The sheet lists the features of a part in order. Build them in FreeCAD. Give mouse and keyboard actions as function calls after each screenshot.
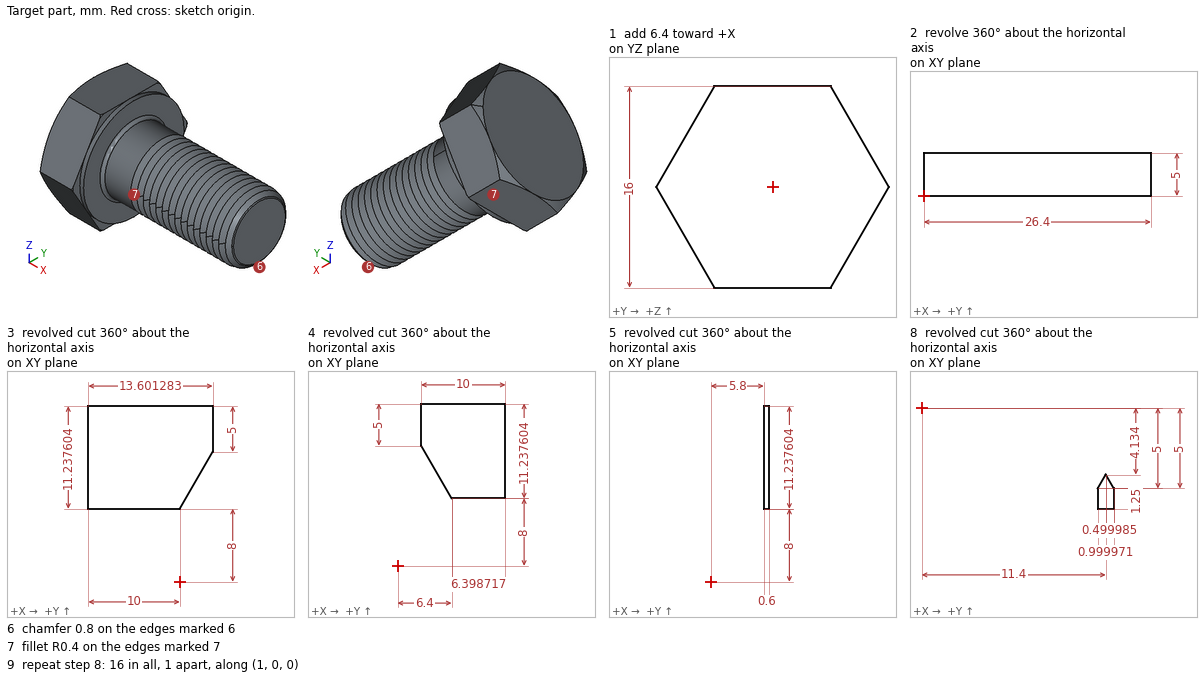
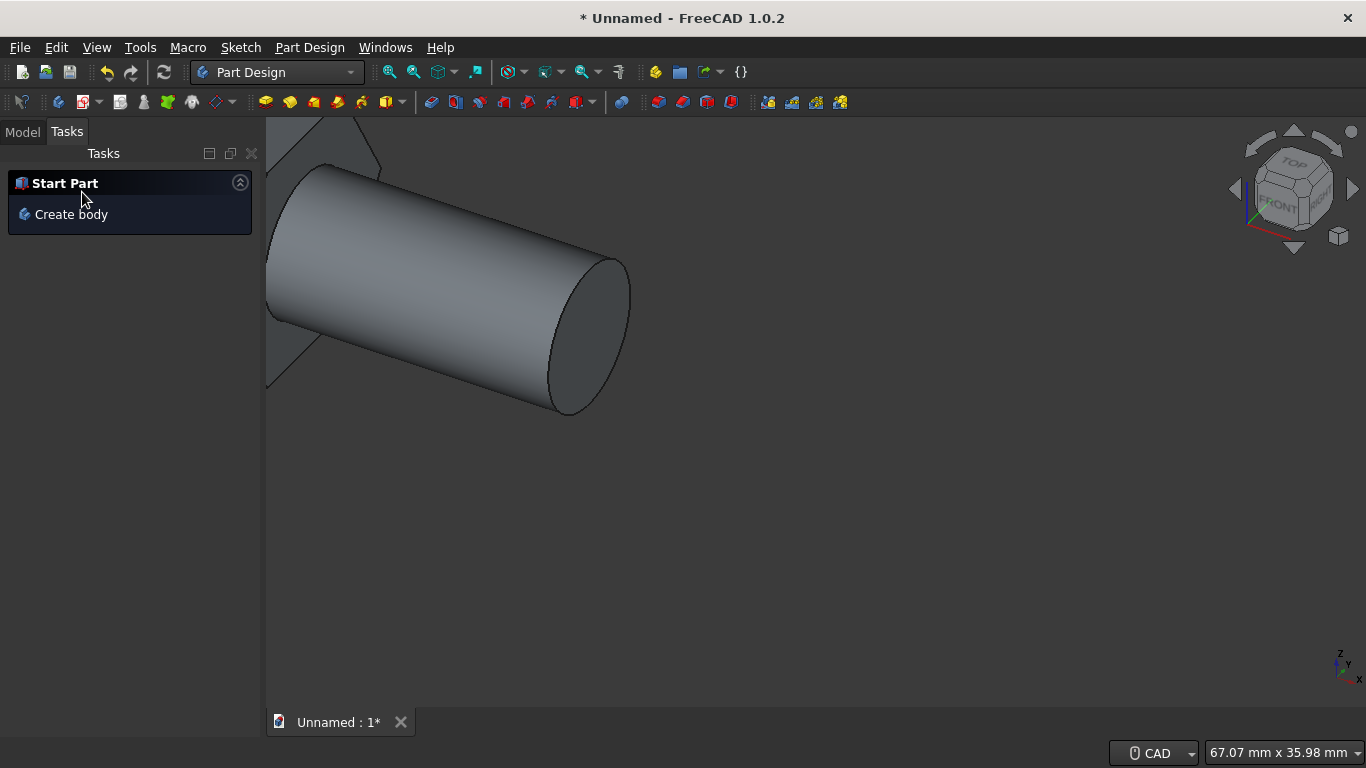
key(v)
key(f)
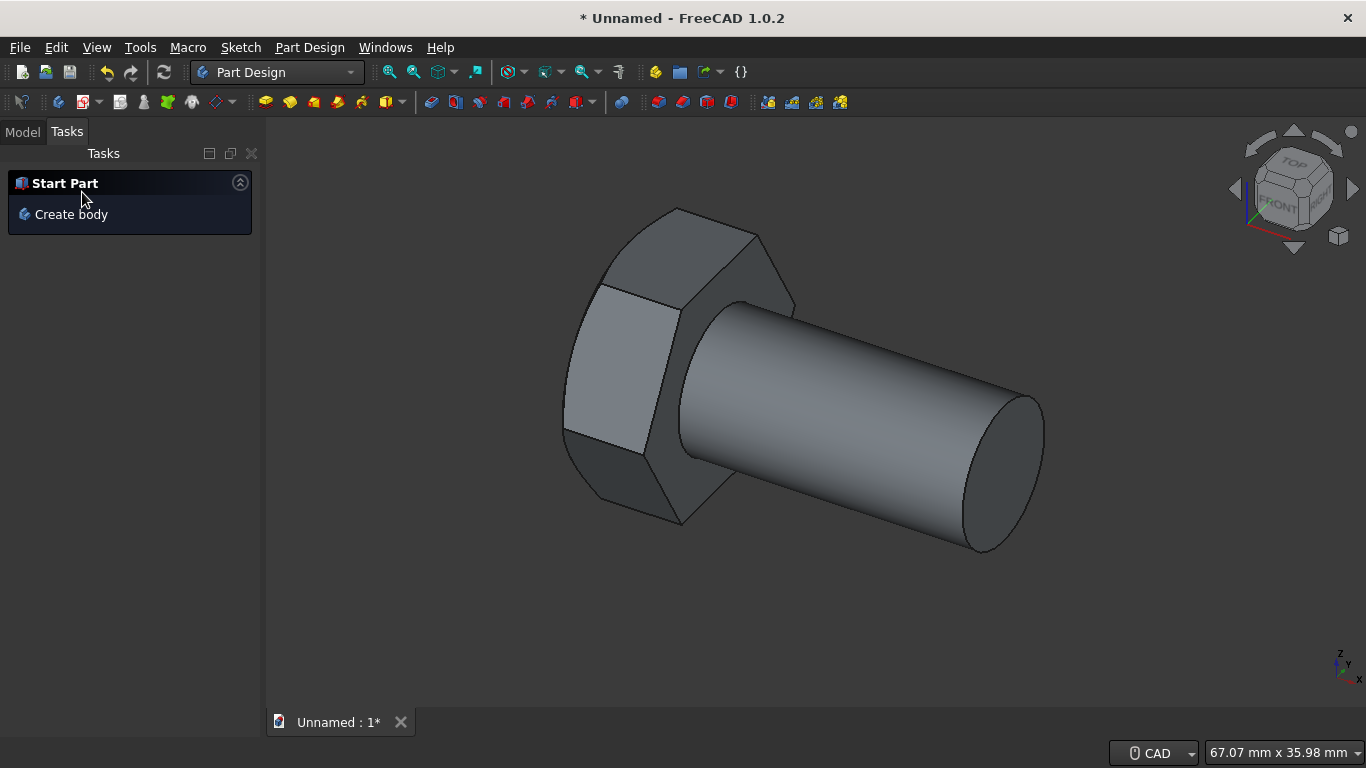
click(84, 102)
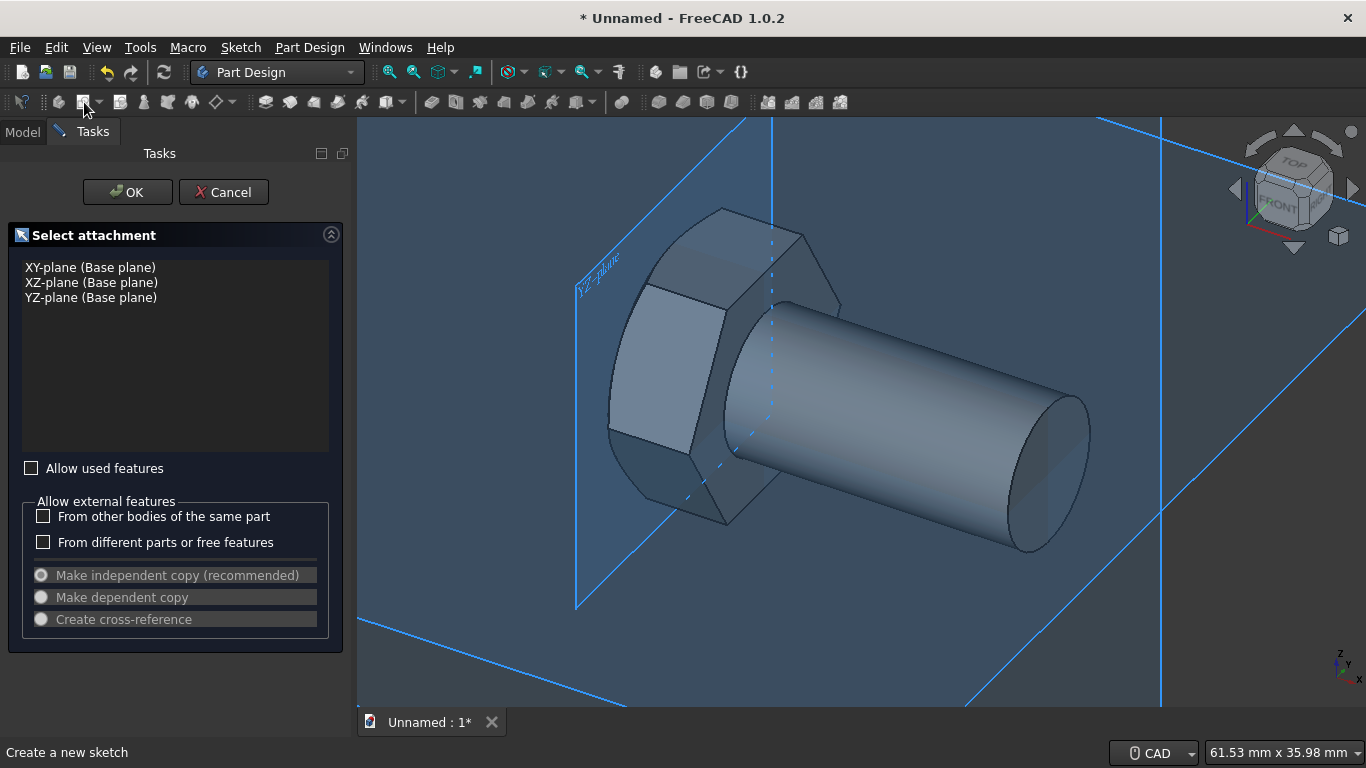
click(82, 268)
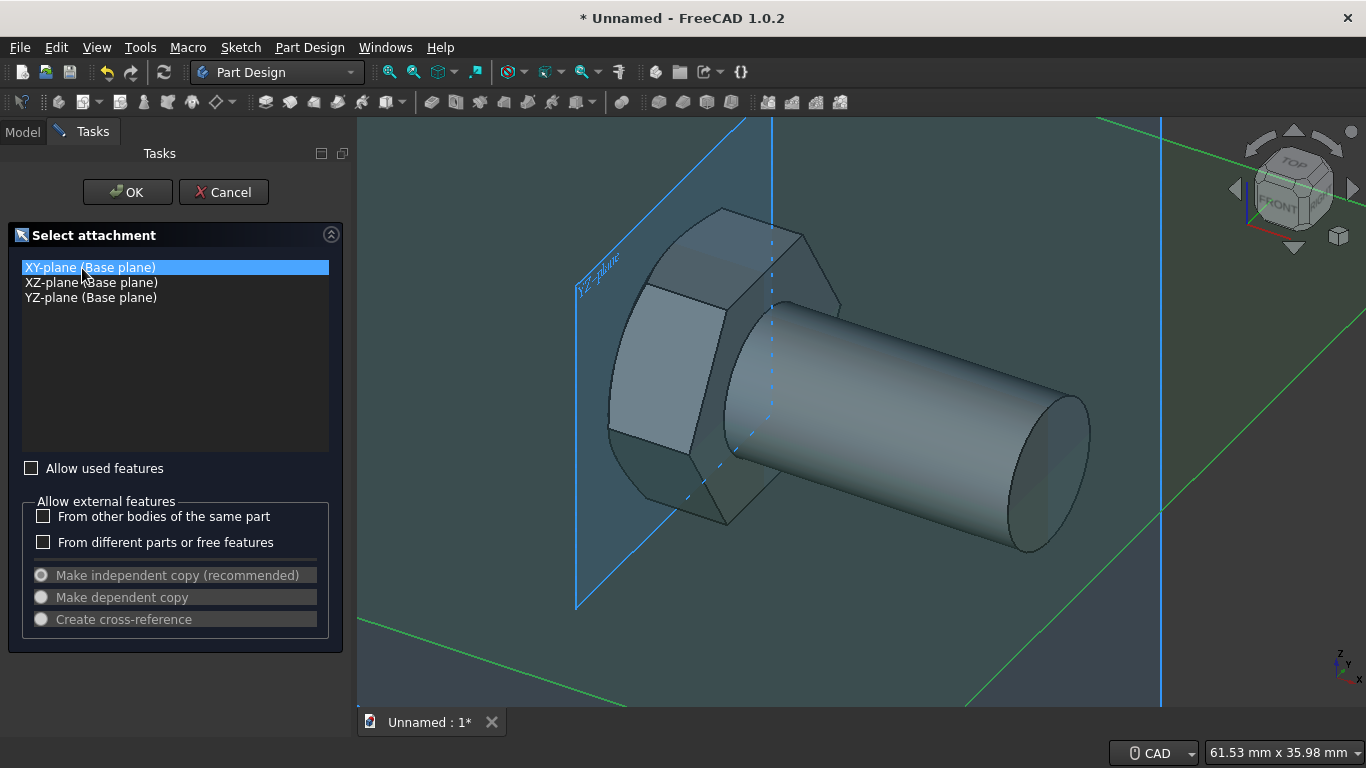
click(128, 192)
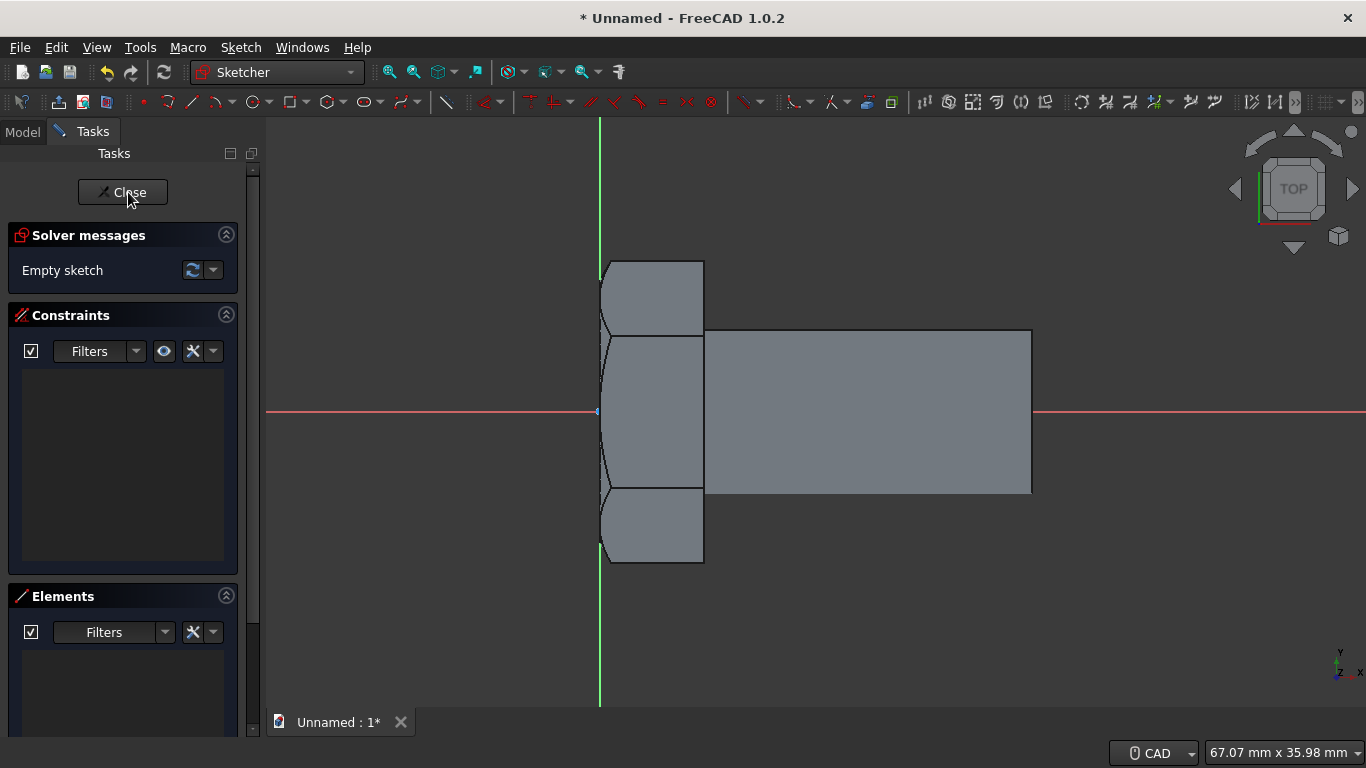
key(q)
key(s)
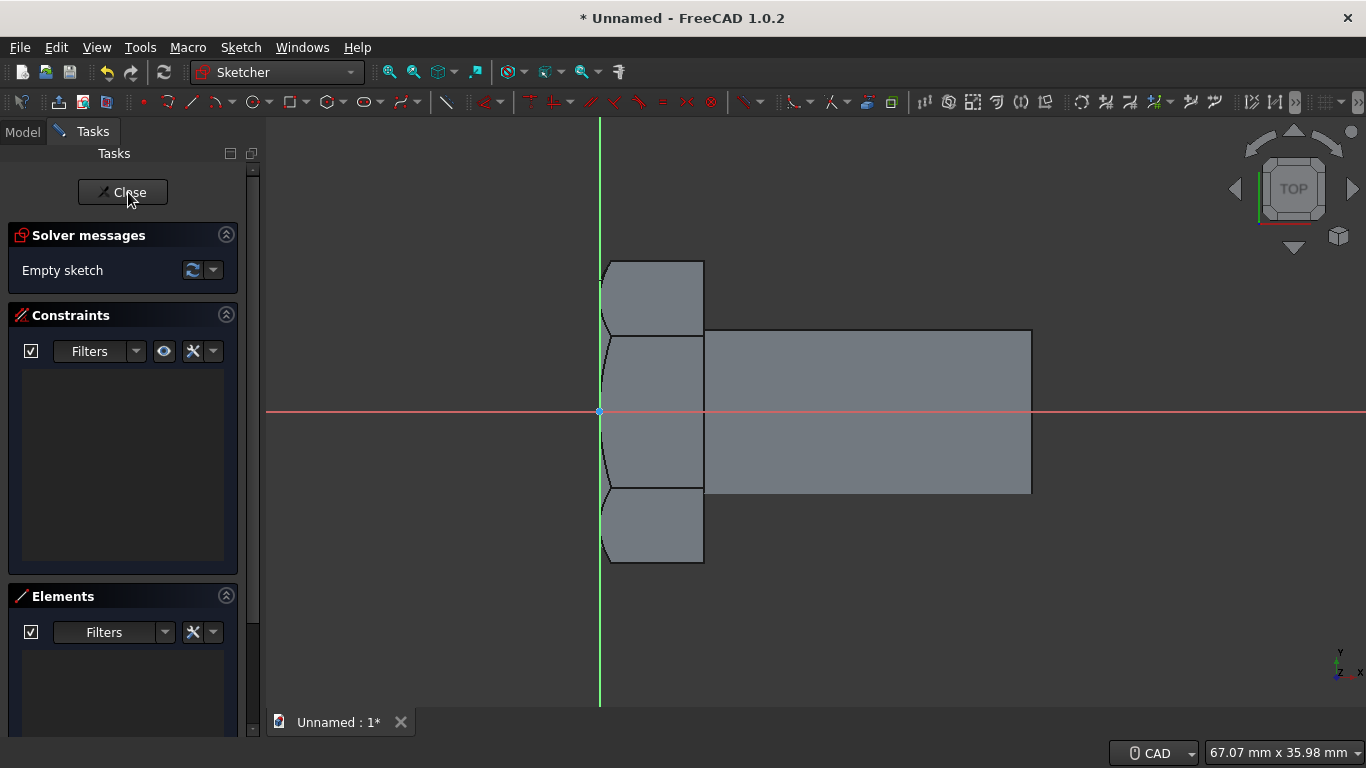
scroll(942, 679, down, 1)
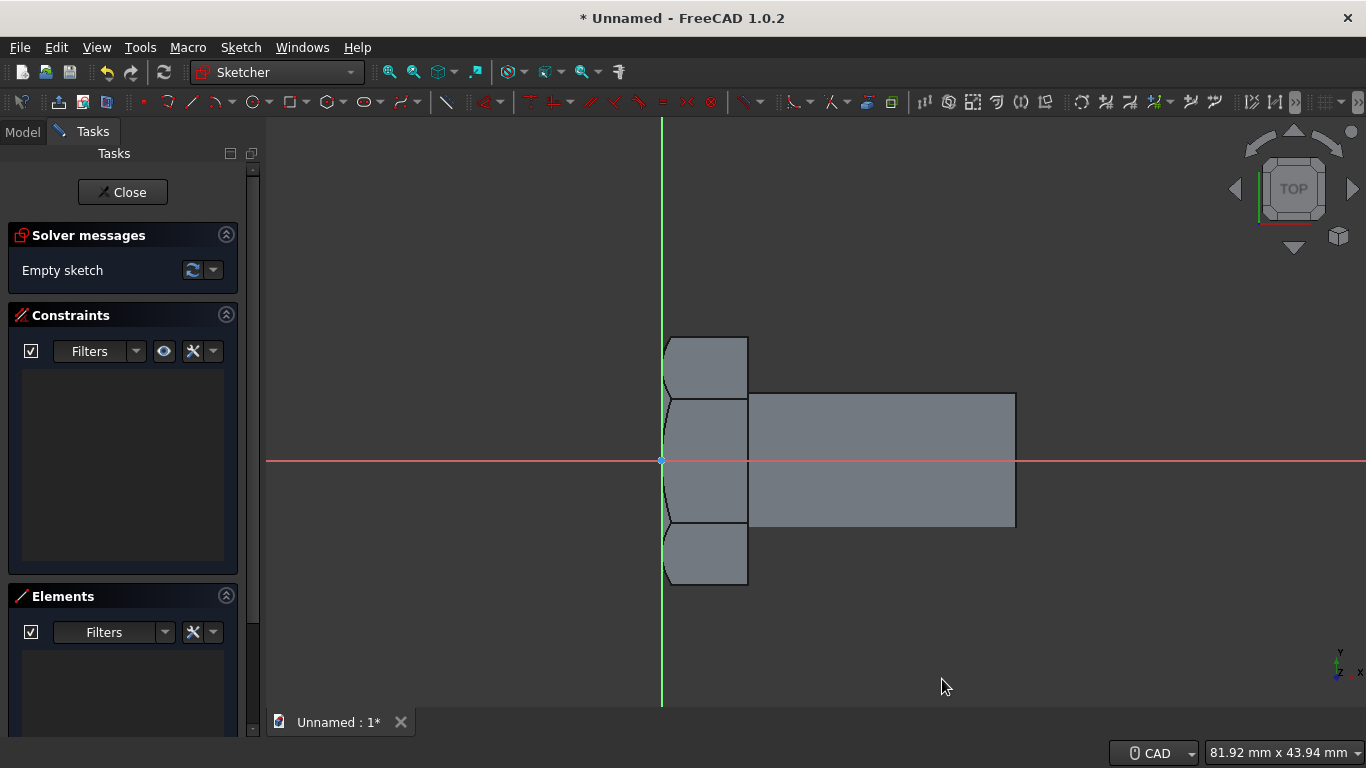
scroll(748, 168, up, 2)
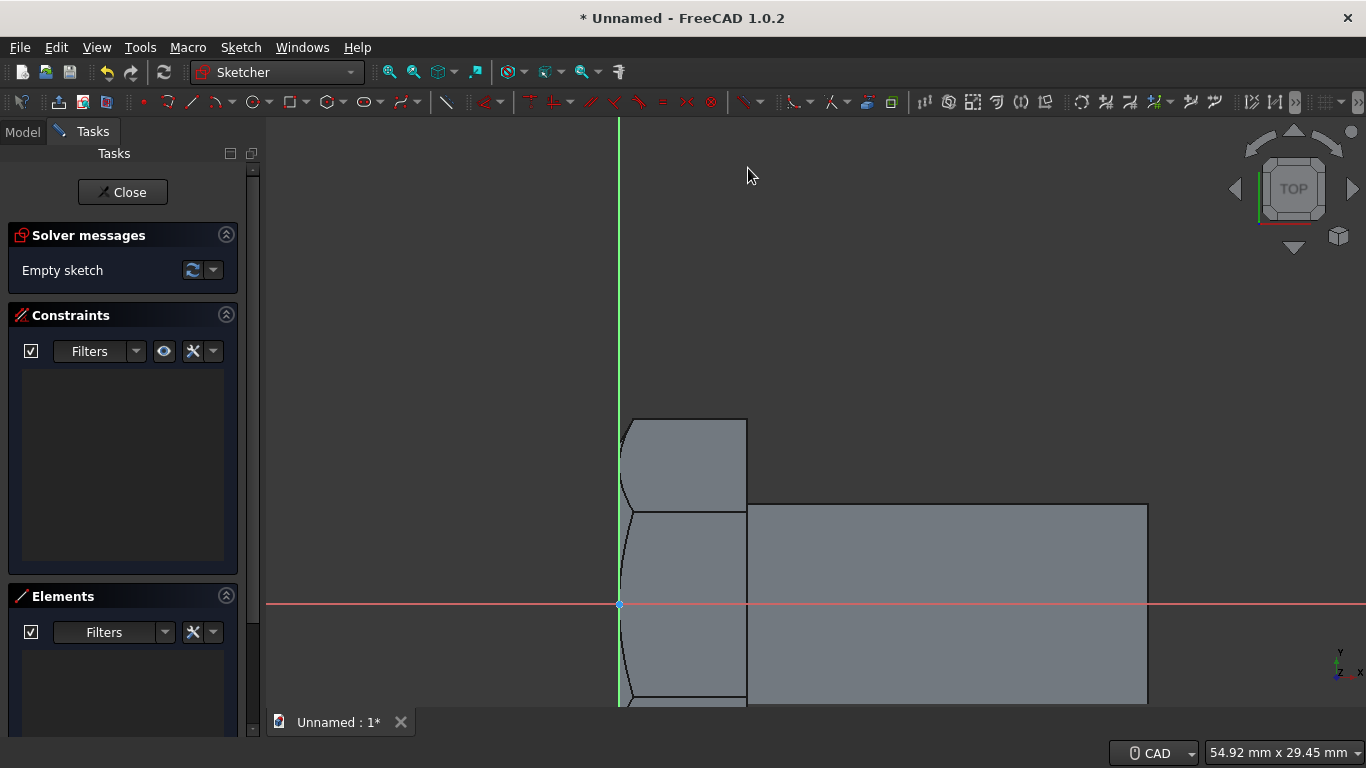
key(g)
key(m)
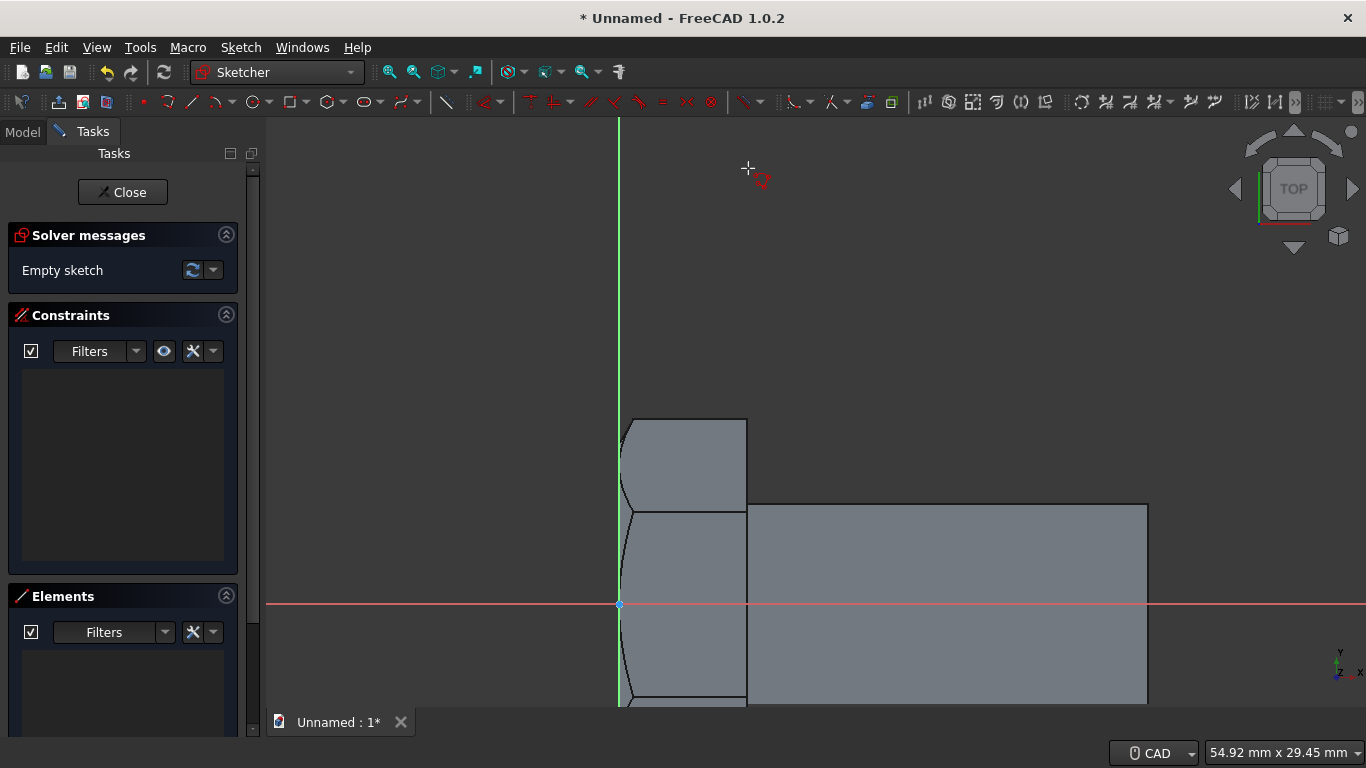
click(747, 444)
click(875, 444)
click(875, 219)
click(675, 219)
click(675, 319)
click(747, 445)
key(Escape)
key(Escape)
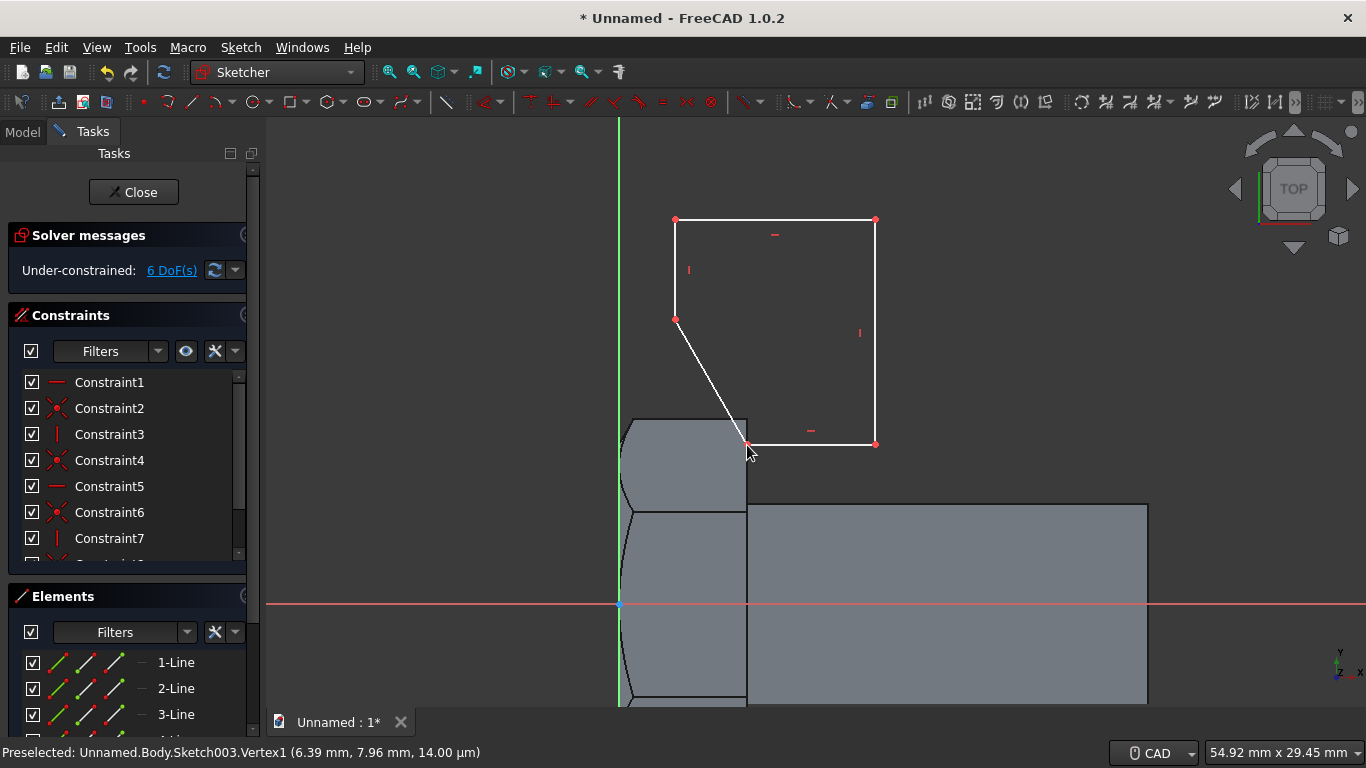
key(d)